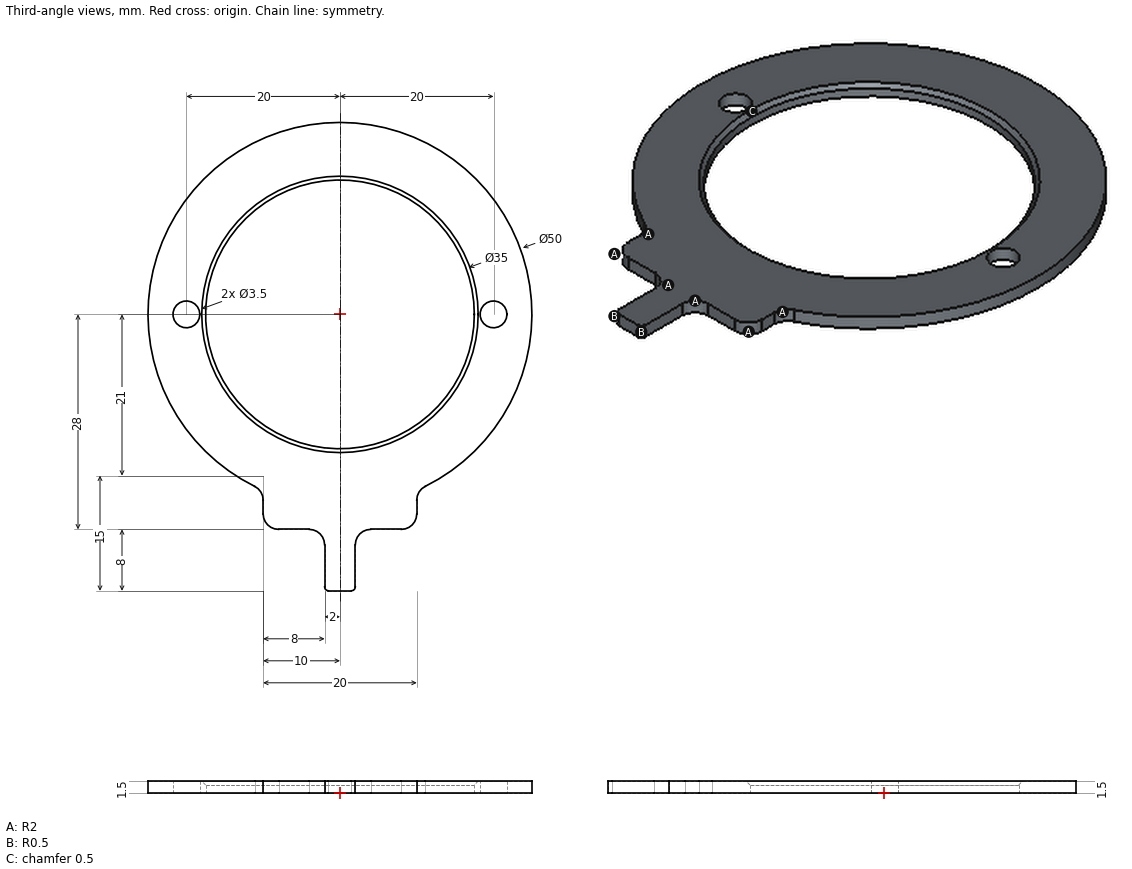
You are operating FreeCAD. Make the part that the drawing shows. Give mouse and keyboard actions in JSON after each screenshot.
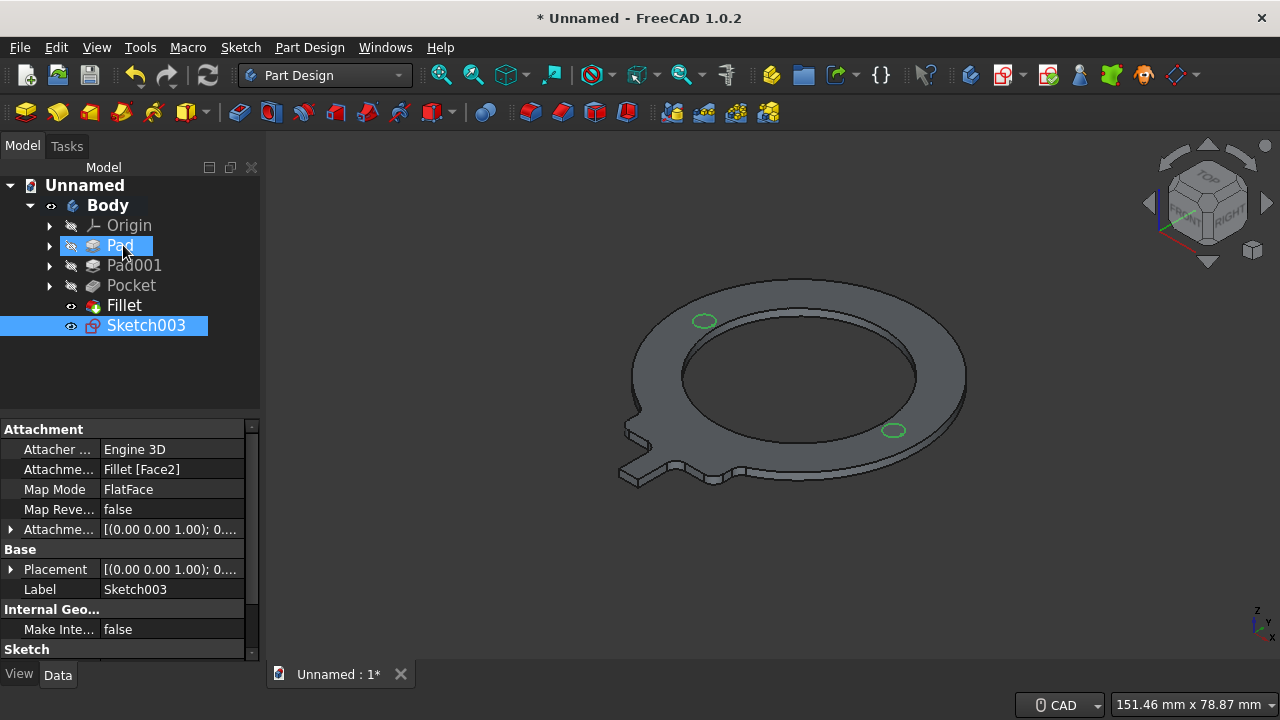
{"action": "left_click", "coordinate": [240, 112]}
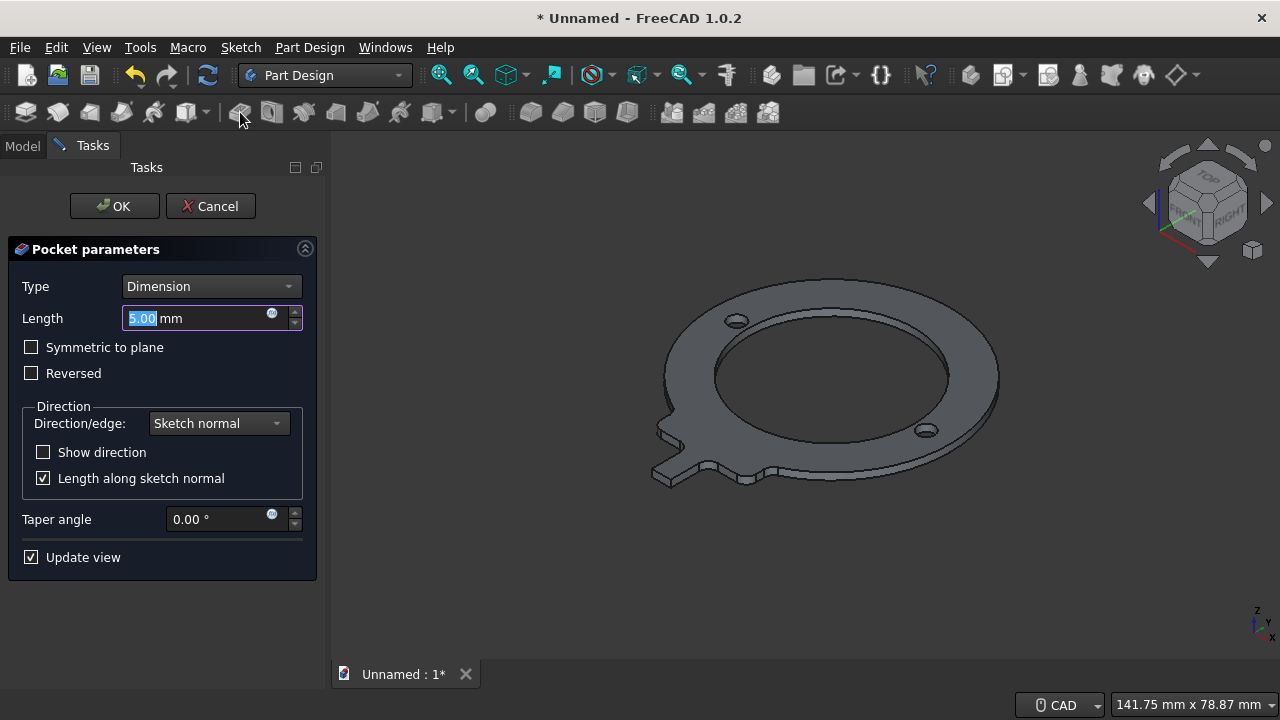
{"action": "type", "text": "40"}
{"action": "key", "text": "Tab"}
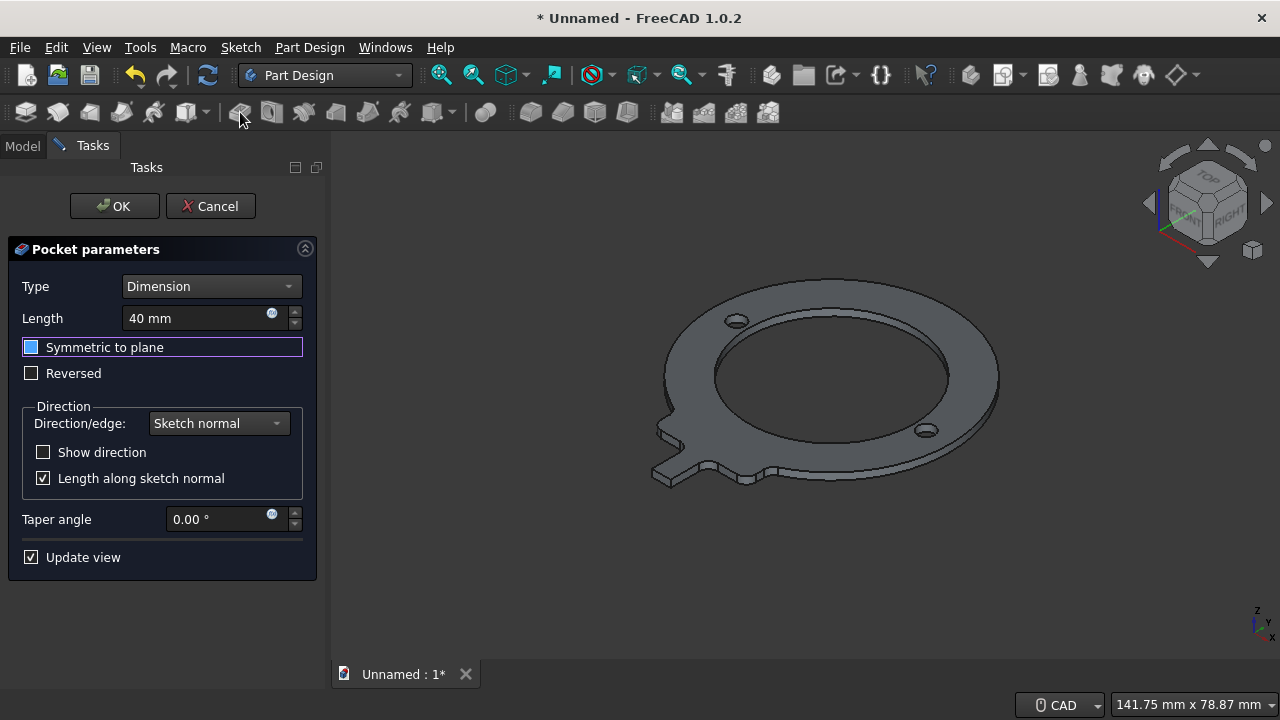
{"action": "left_click", "coordinate": [115, 206]}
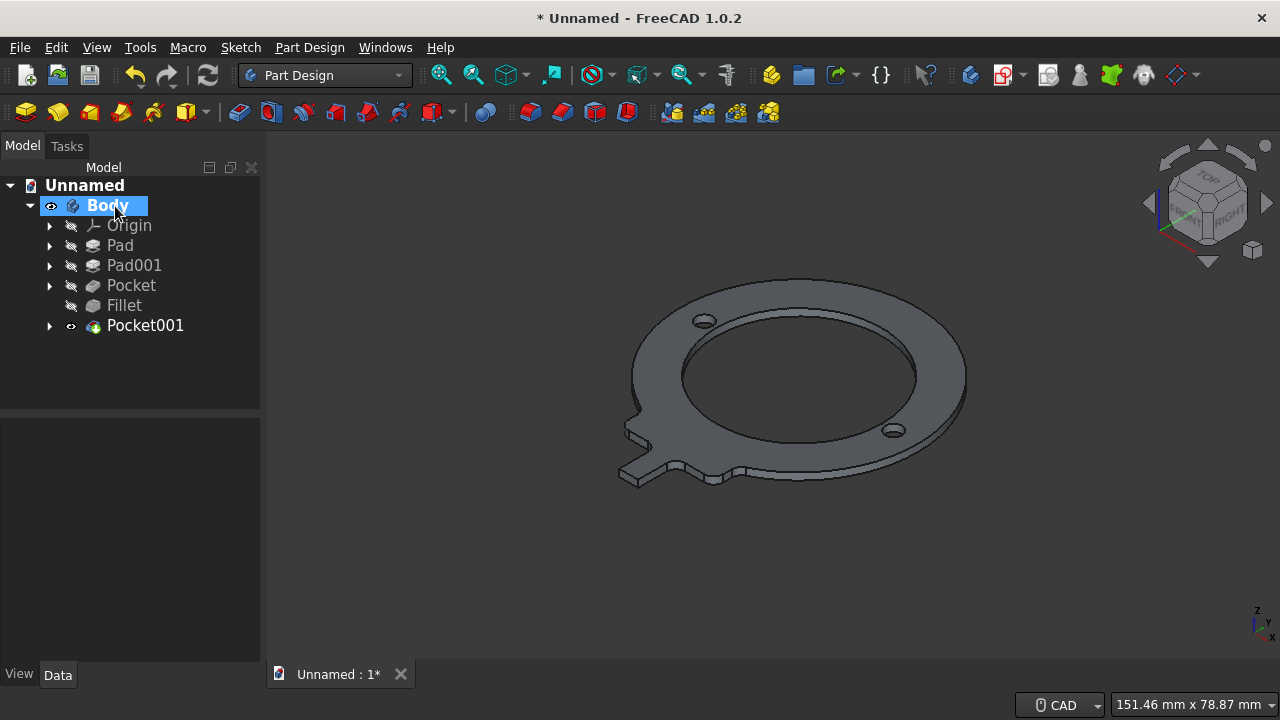
{"action": "scroll", "coordinate": [619, 472], "scroll_direction": "up", "scroll_amount": 7}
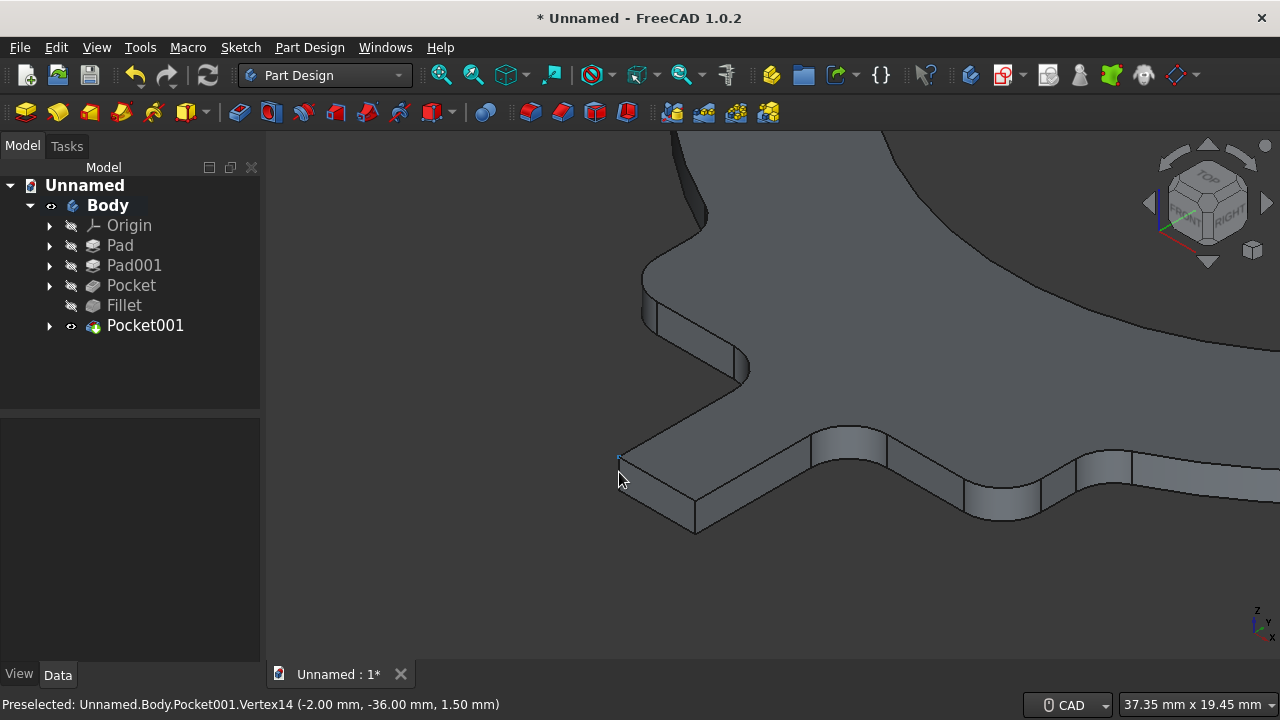
{"action": "left_click", "coordinate": [695, 517]}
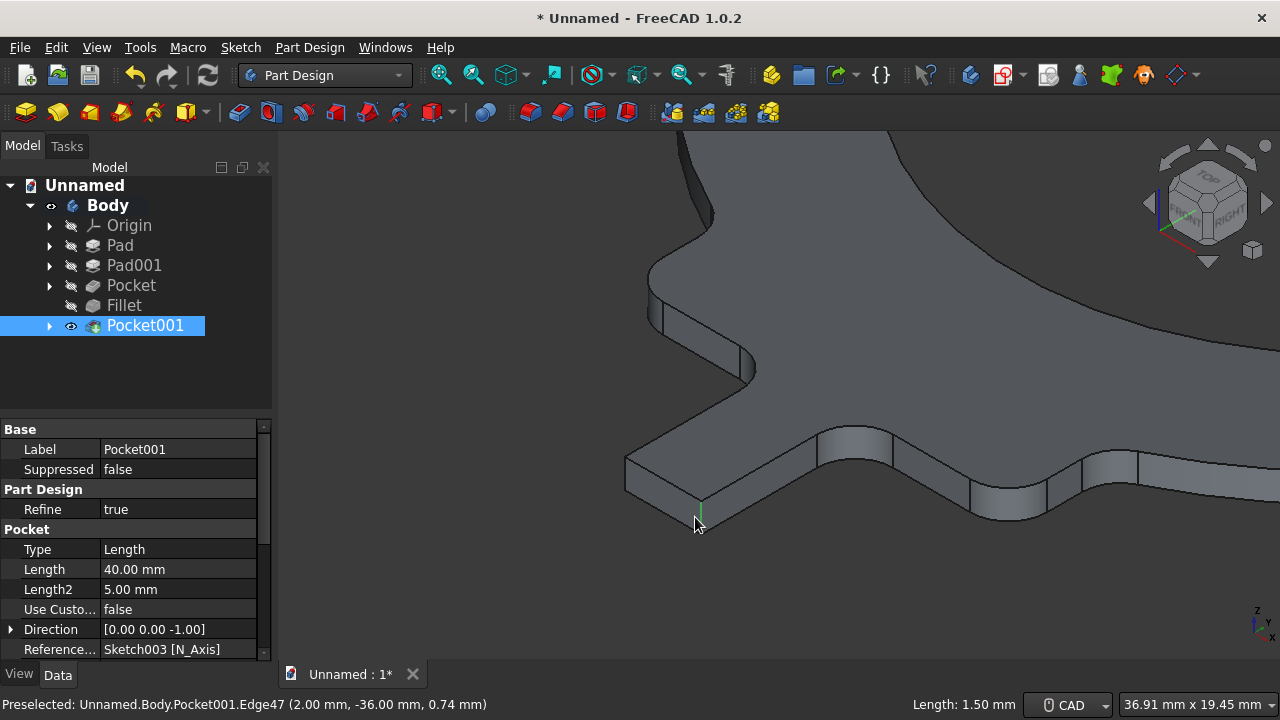
{"action": "left_click", "coordinate": [442, 76]}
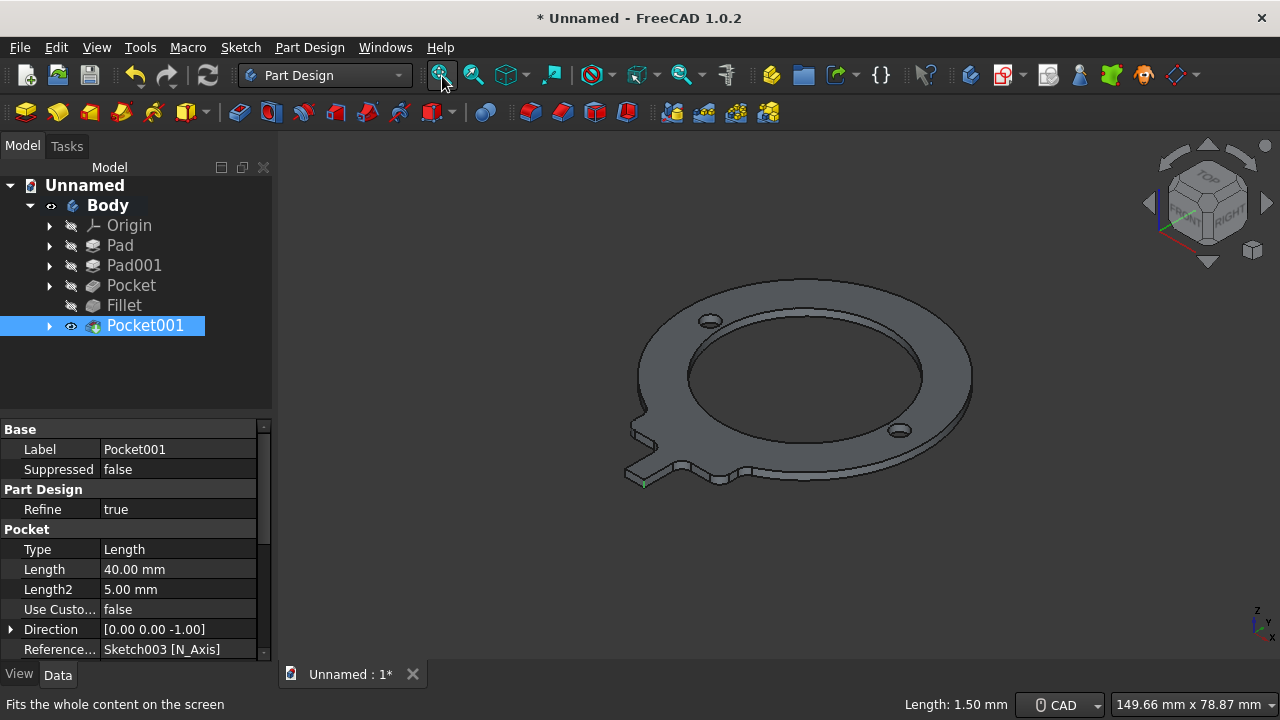
{"action": "key", "text": "2"}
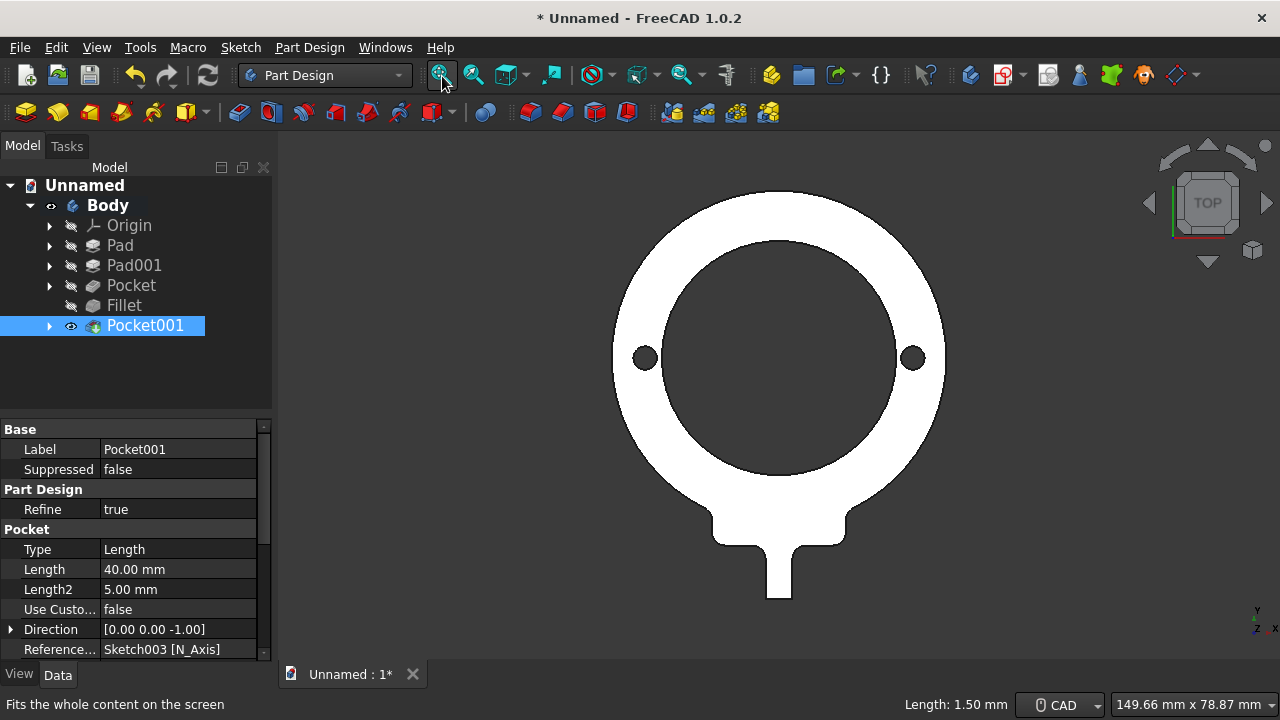
{"action": "scroll", "coordinate": [766, 598], "scroll_direction": "up", "scroll_amount": 7}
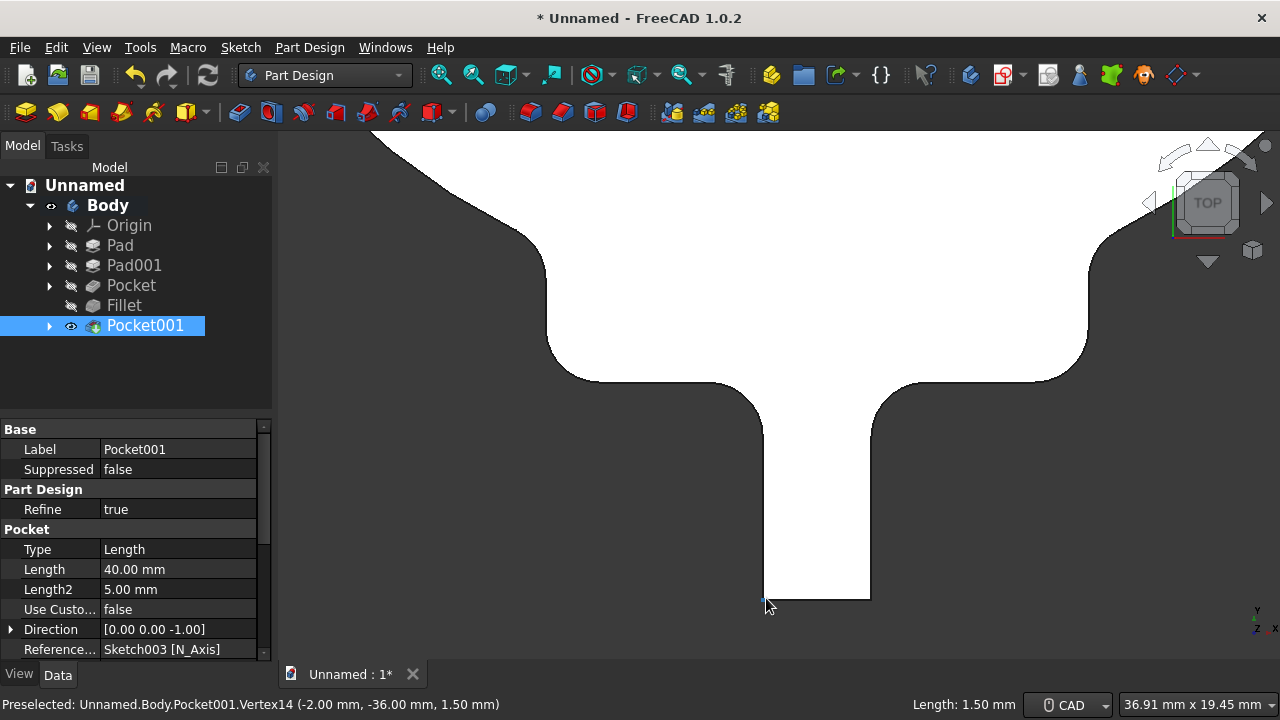
{"action": "left_click", "coordinate": [442, 76]}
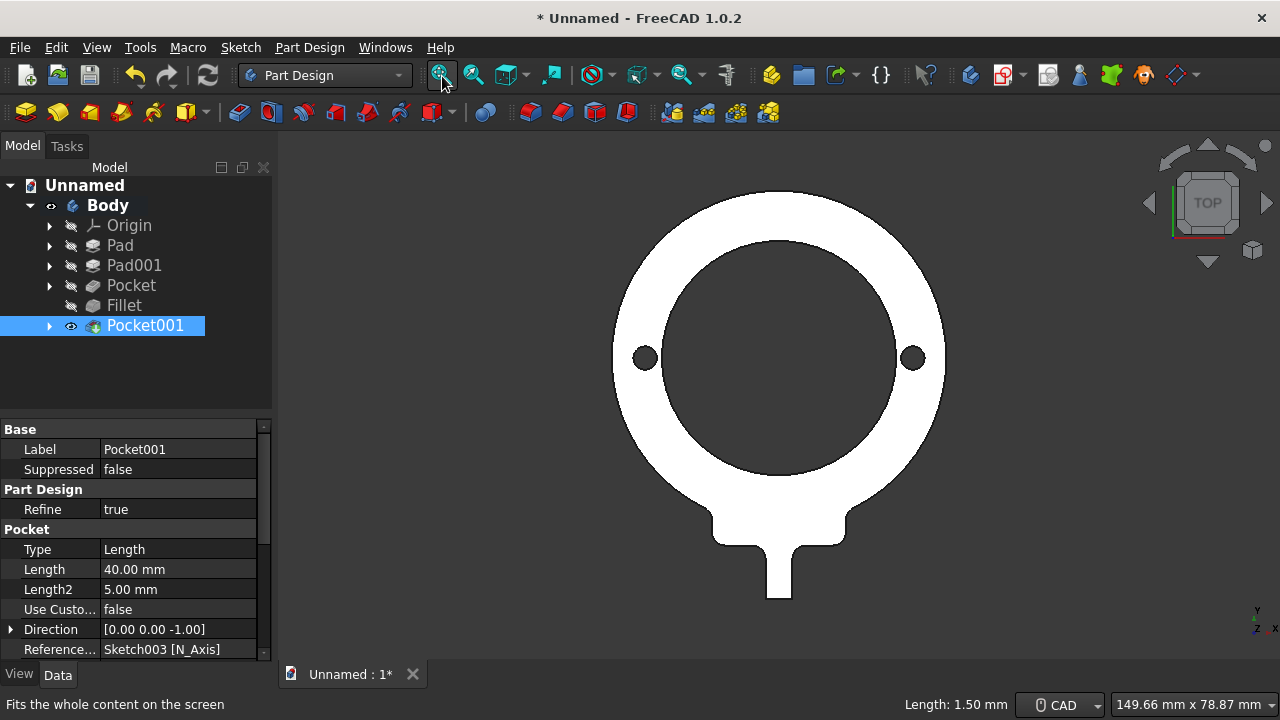
{"action": "key", "text": "0"}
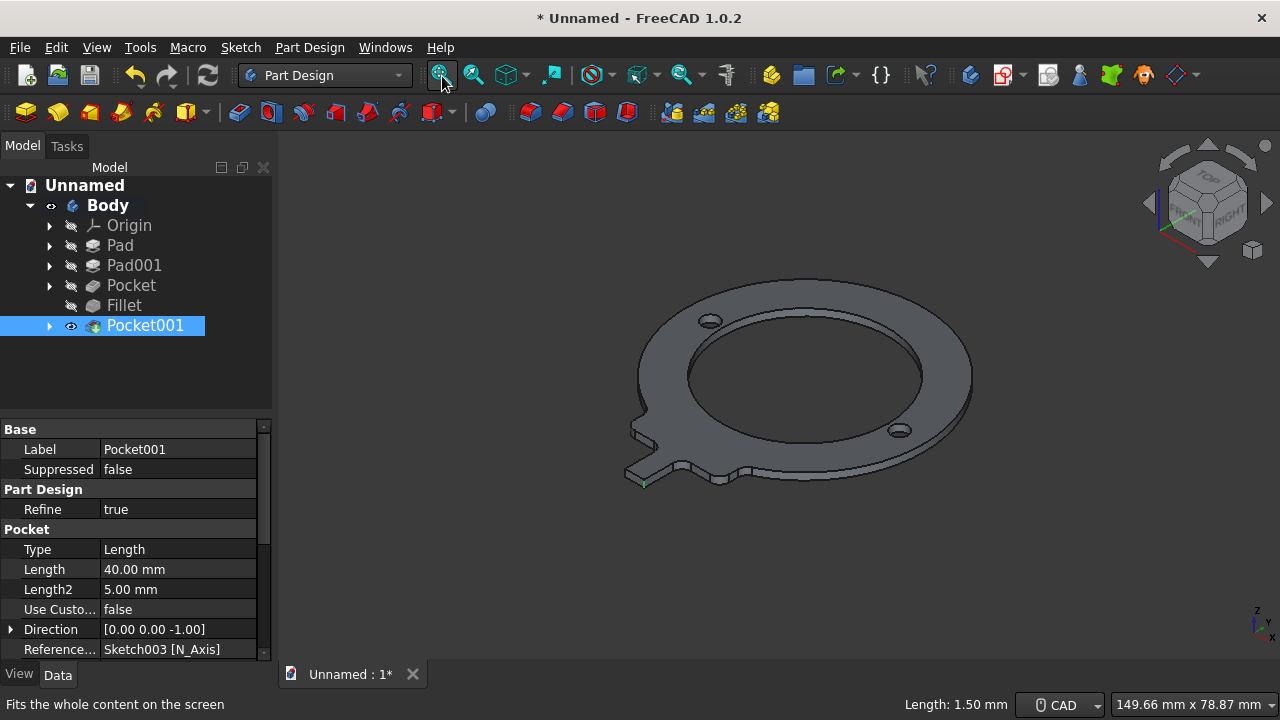
{"action": "scroll", "coordinate": [625, 472], "scroll_direction": "up", "scroll_amount": 7}